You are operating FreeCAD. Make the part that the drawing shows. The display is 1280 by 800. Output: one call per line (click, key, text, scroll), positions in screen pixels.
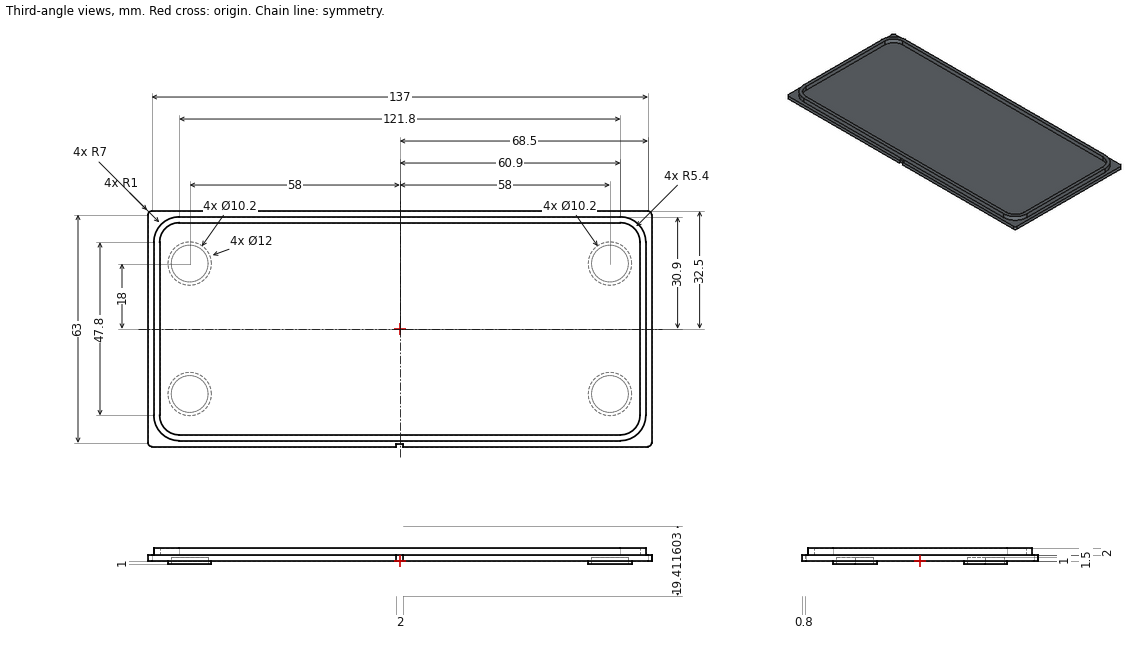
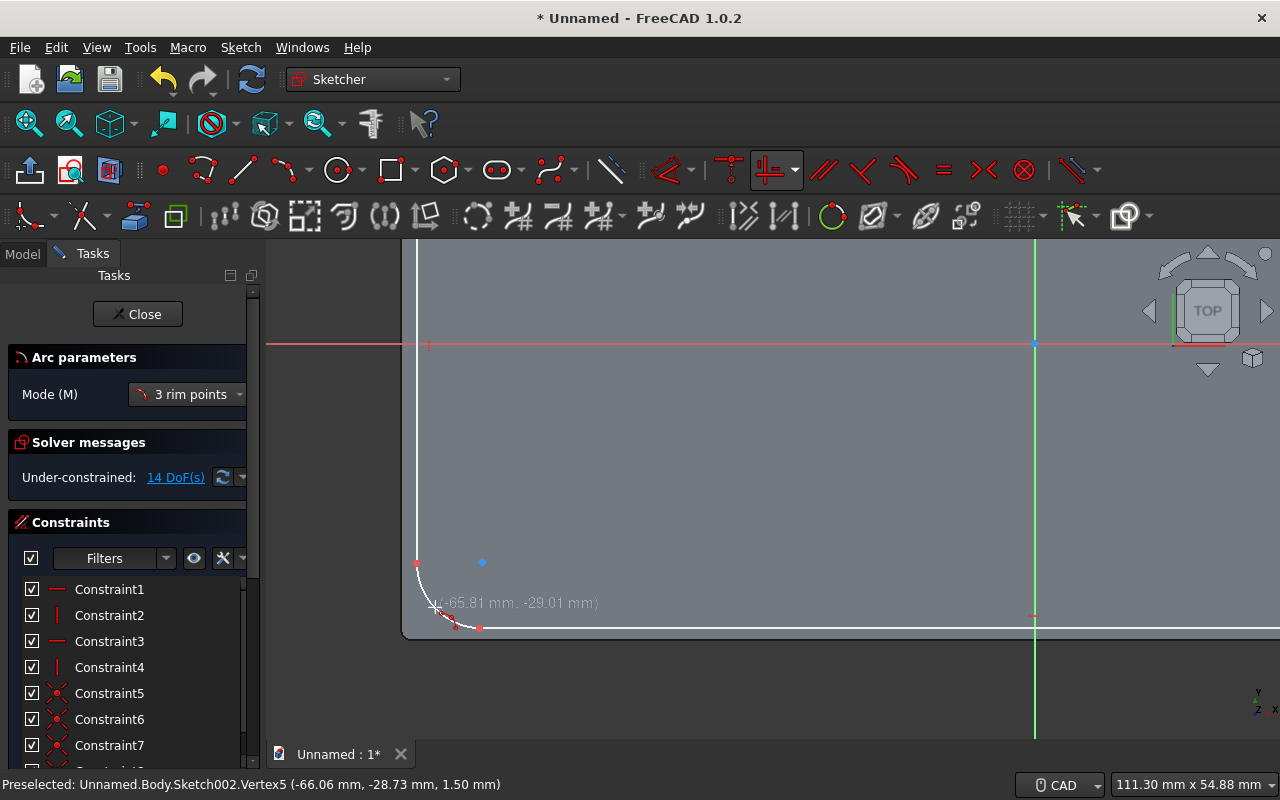
scroll(435, 608, down, 4)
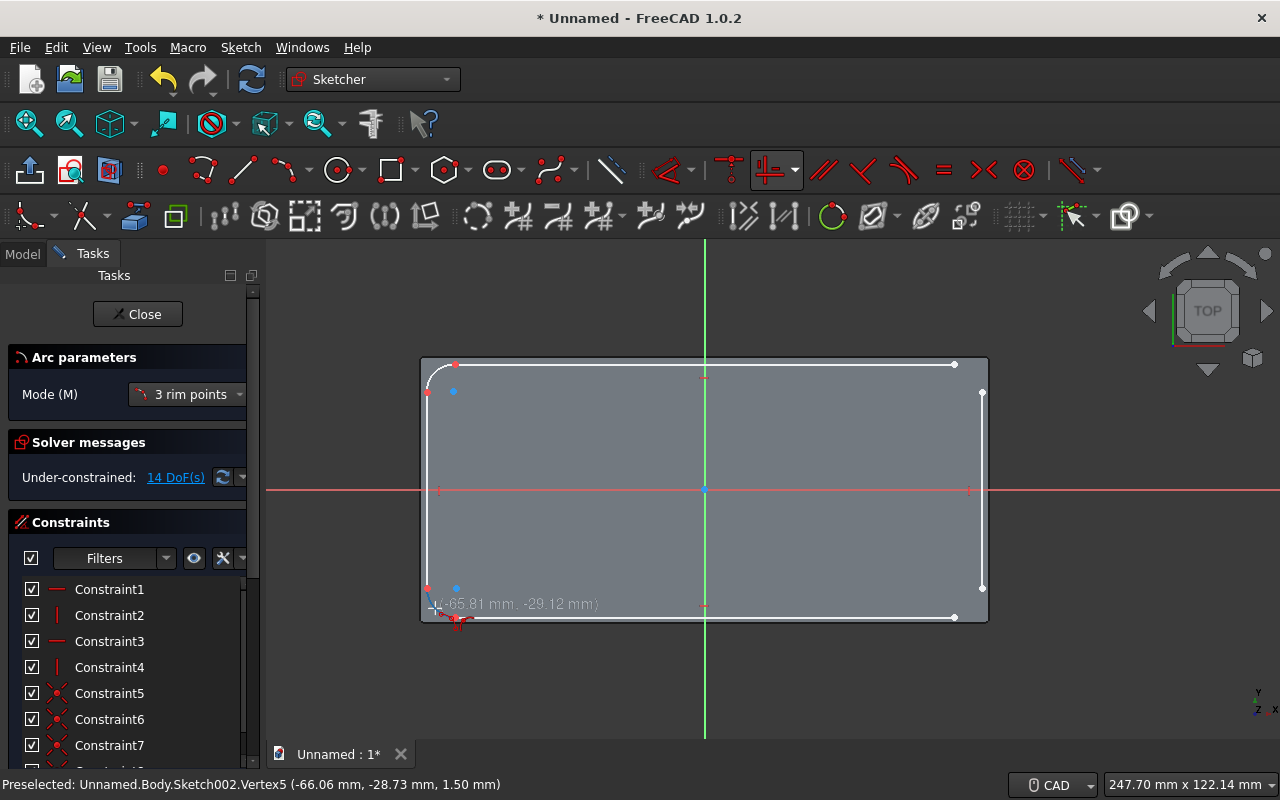
click(954, 618)
click(982, 589)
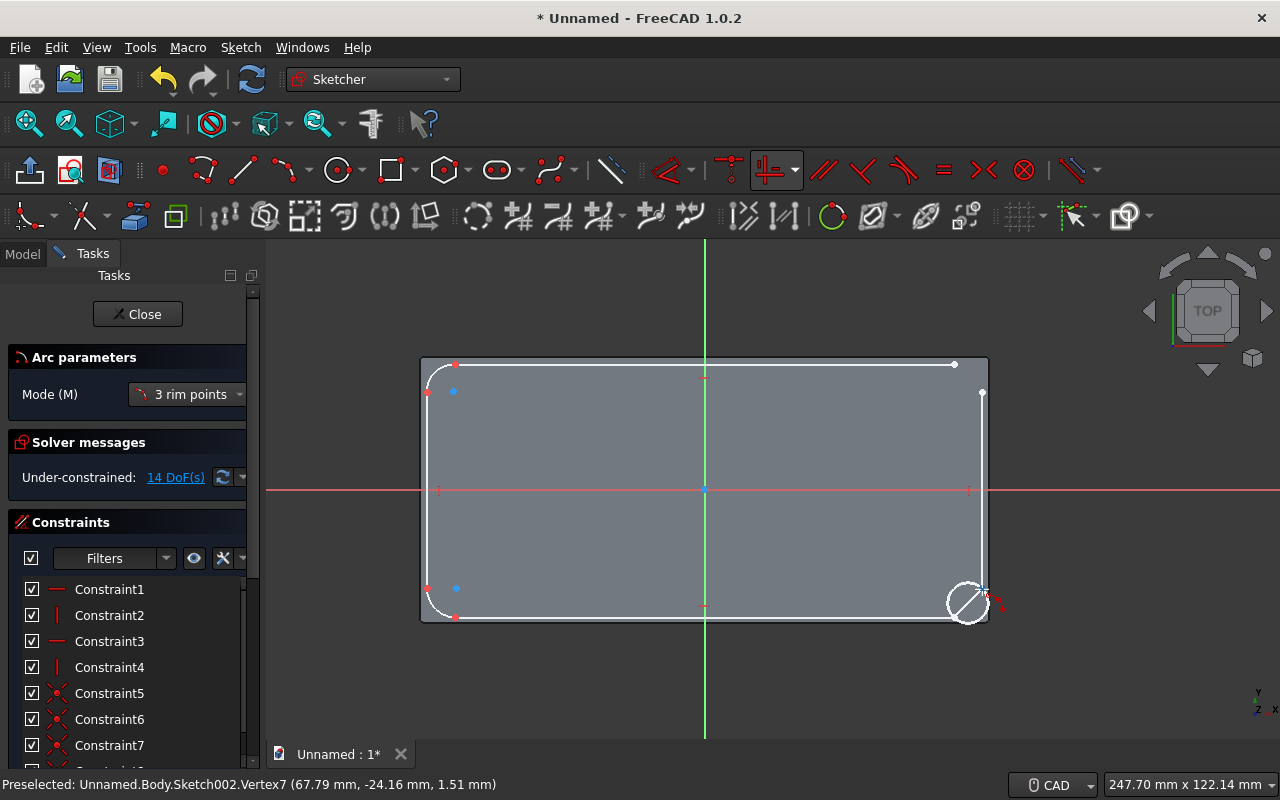
scroll(974, 608, up, 4)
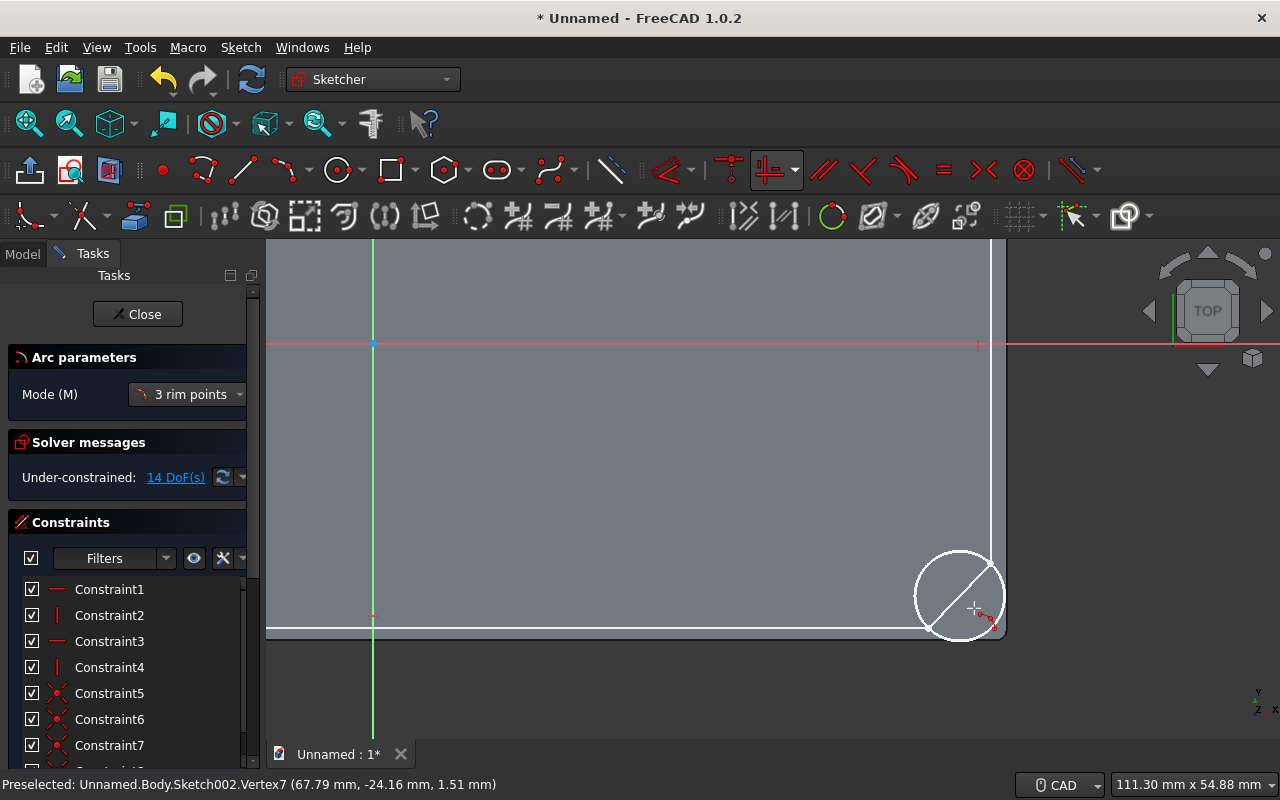
click(973, 607)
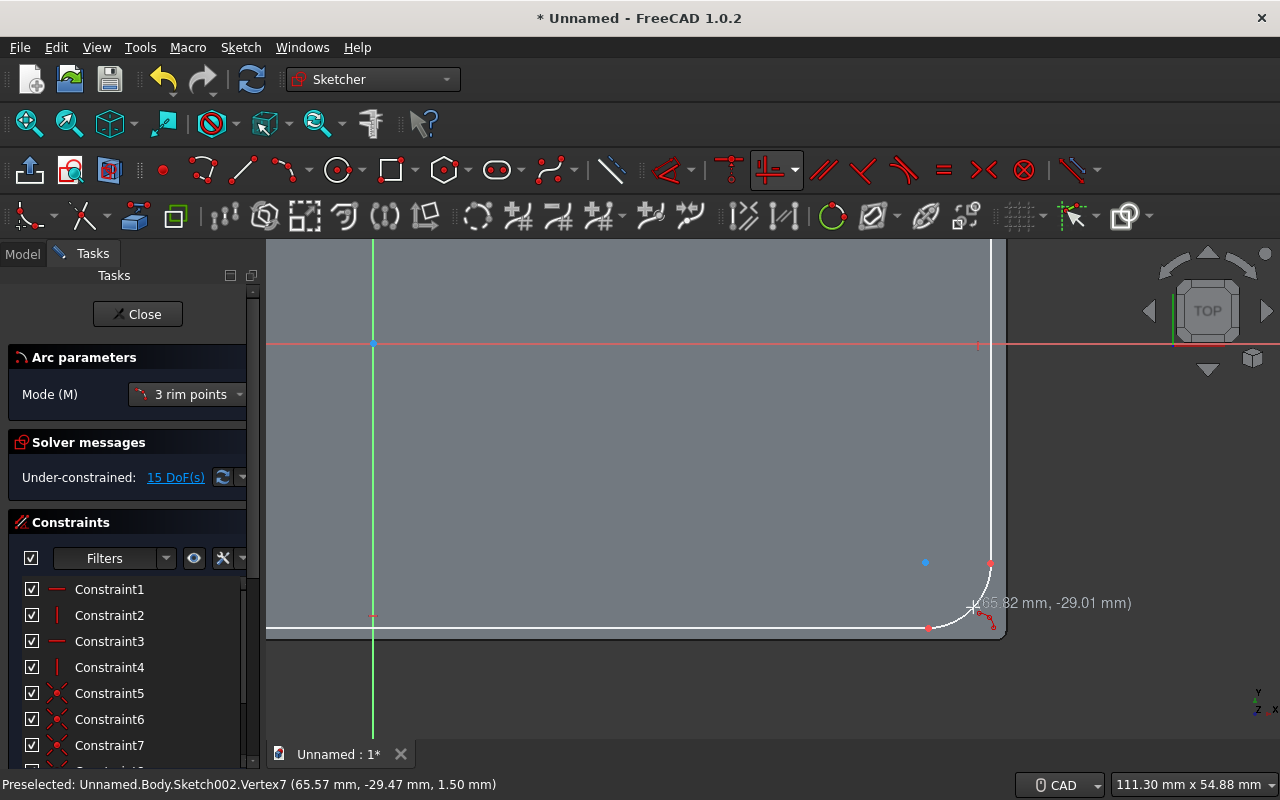
scroll(975, 608, down, 4)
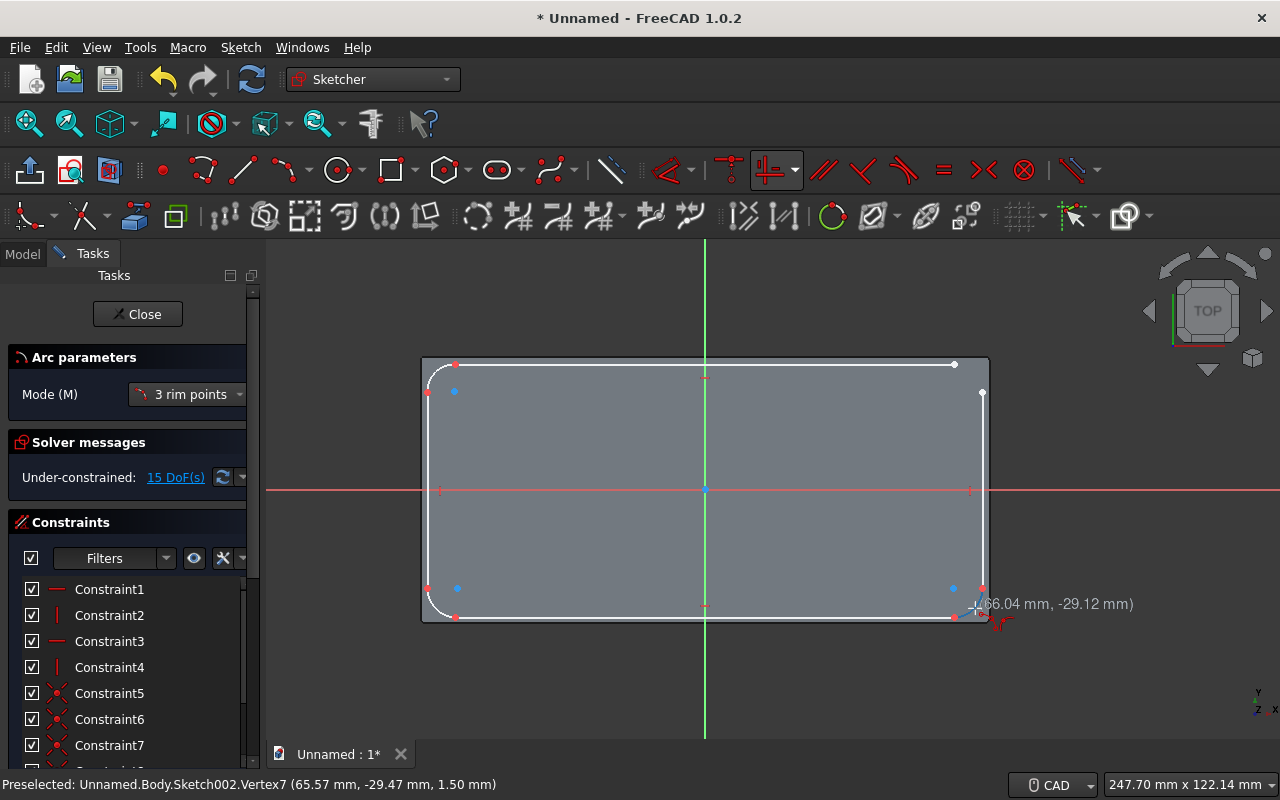
click(983, 393)
click(955, 365)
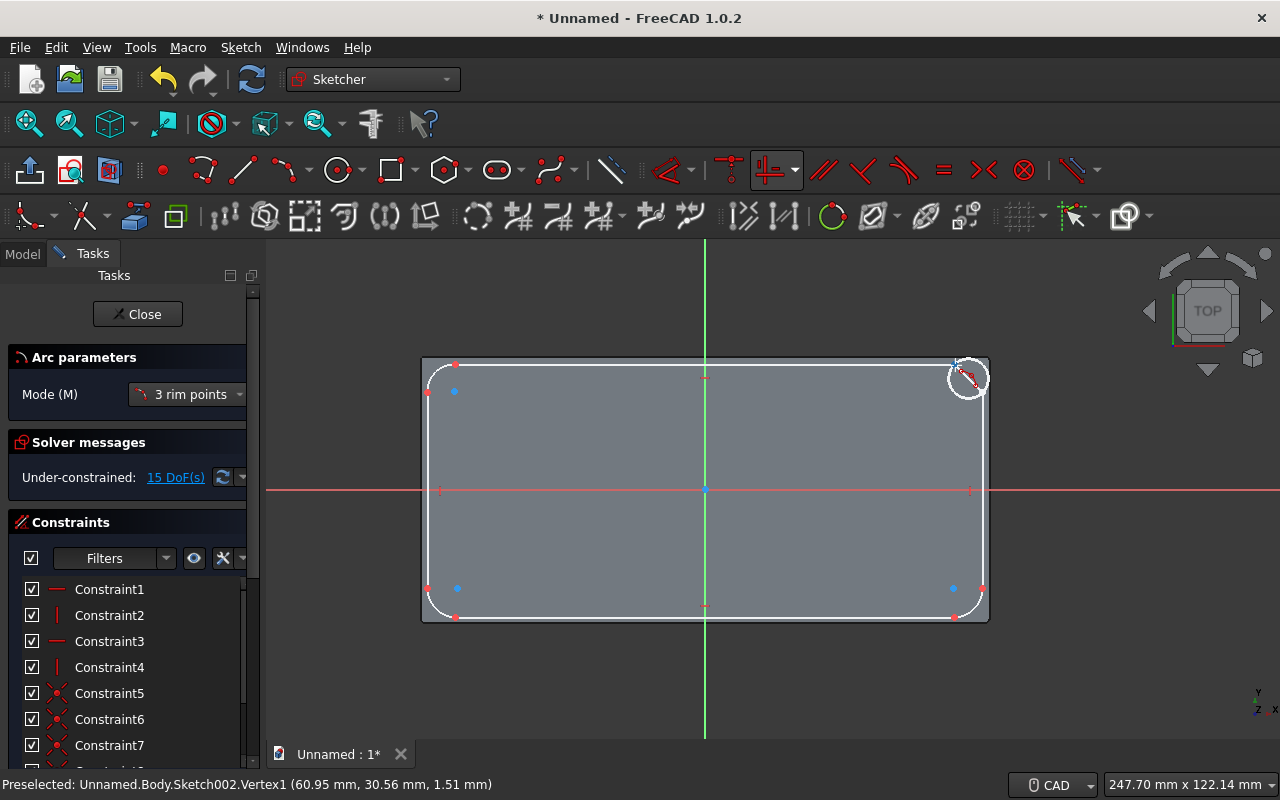
scroll(975, 372, up, 4)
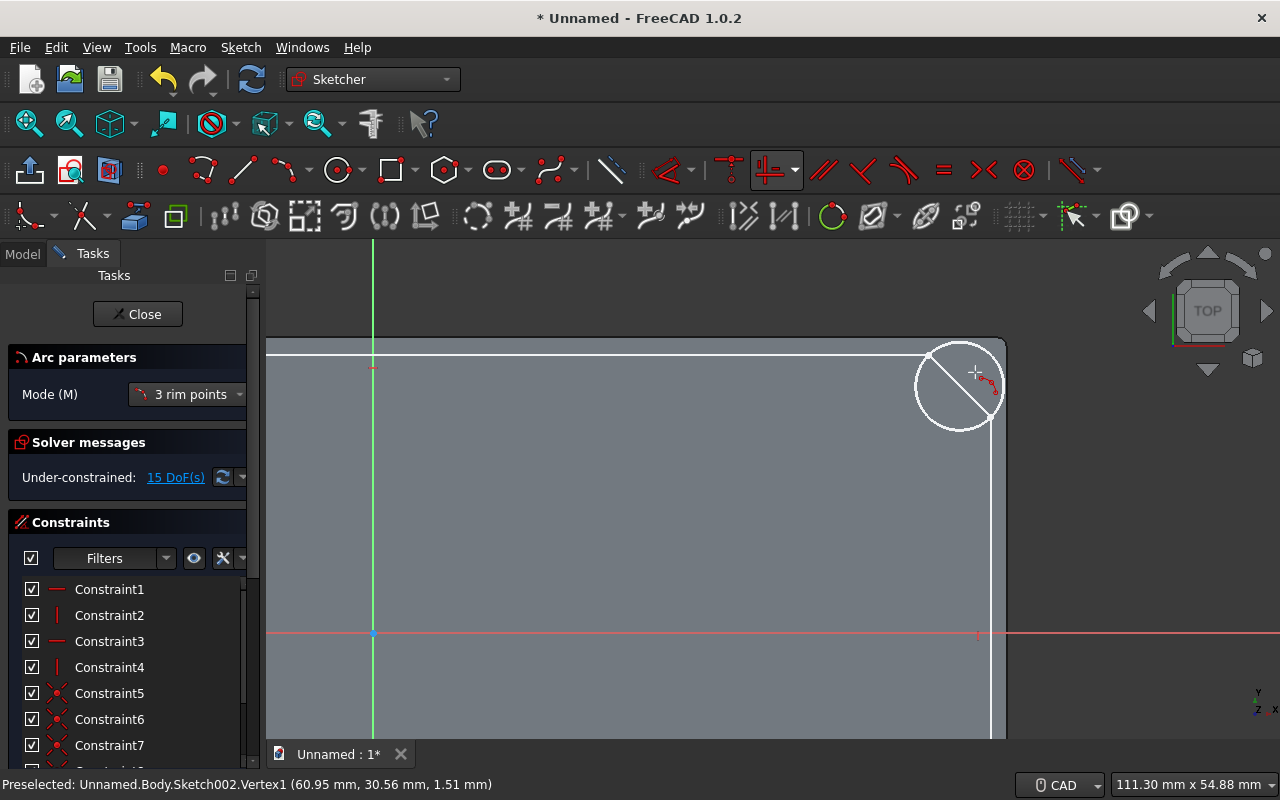
click(973, 371)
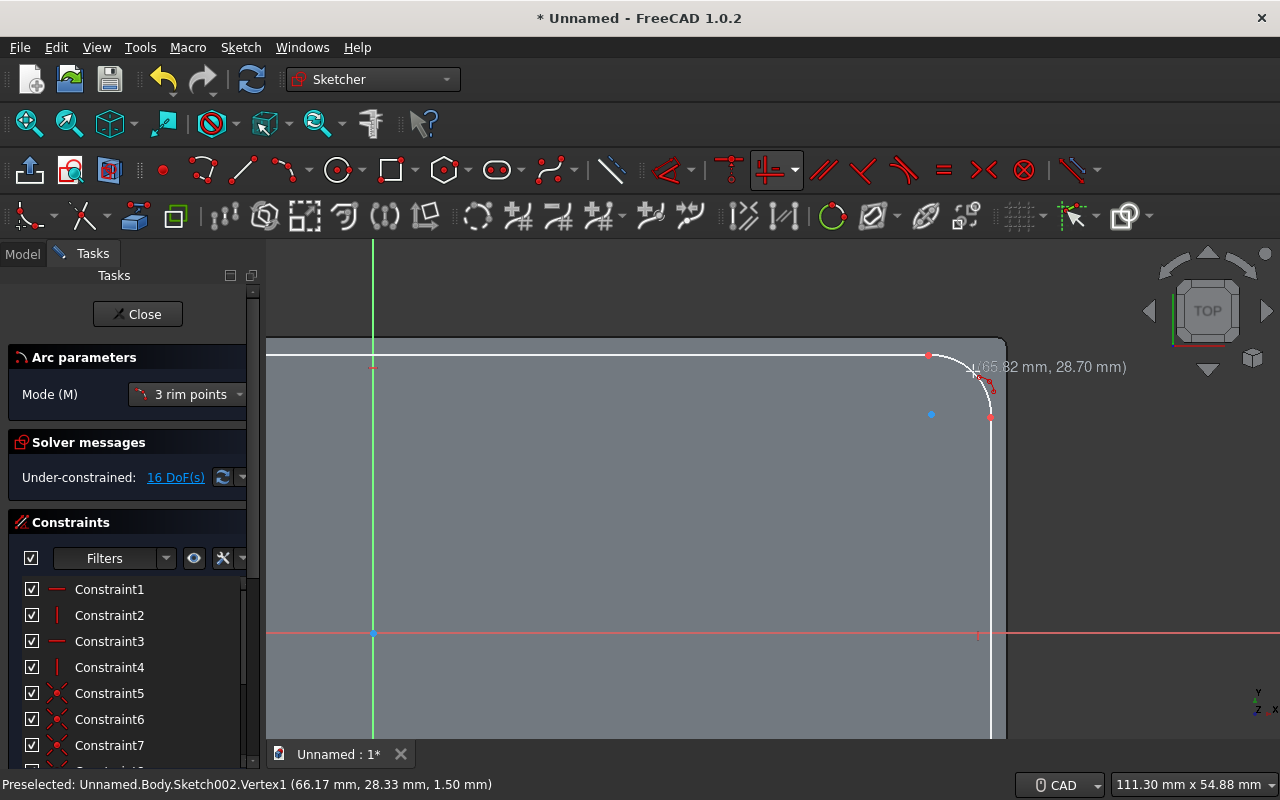
click(244, 170)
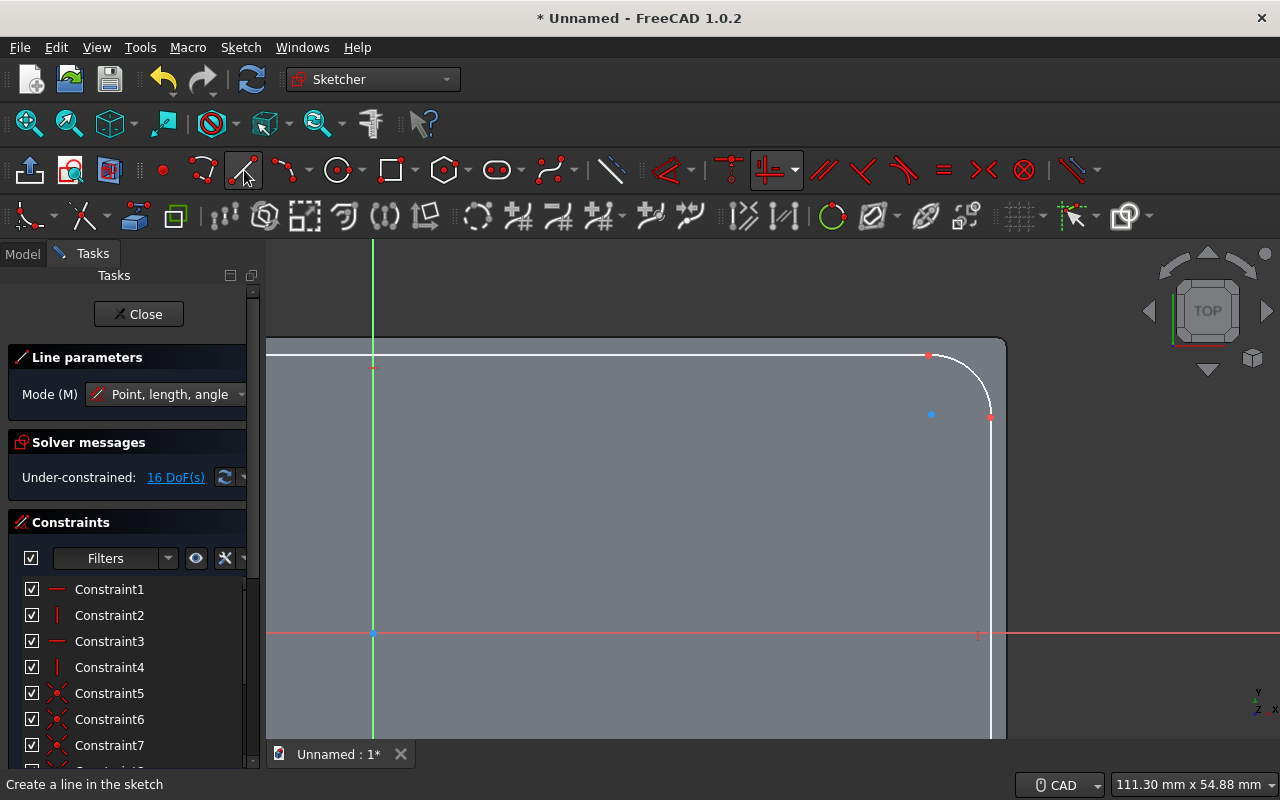
scroll(975, 371, down, 4)